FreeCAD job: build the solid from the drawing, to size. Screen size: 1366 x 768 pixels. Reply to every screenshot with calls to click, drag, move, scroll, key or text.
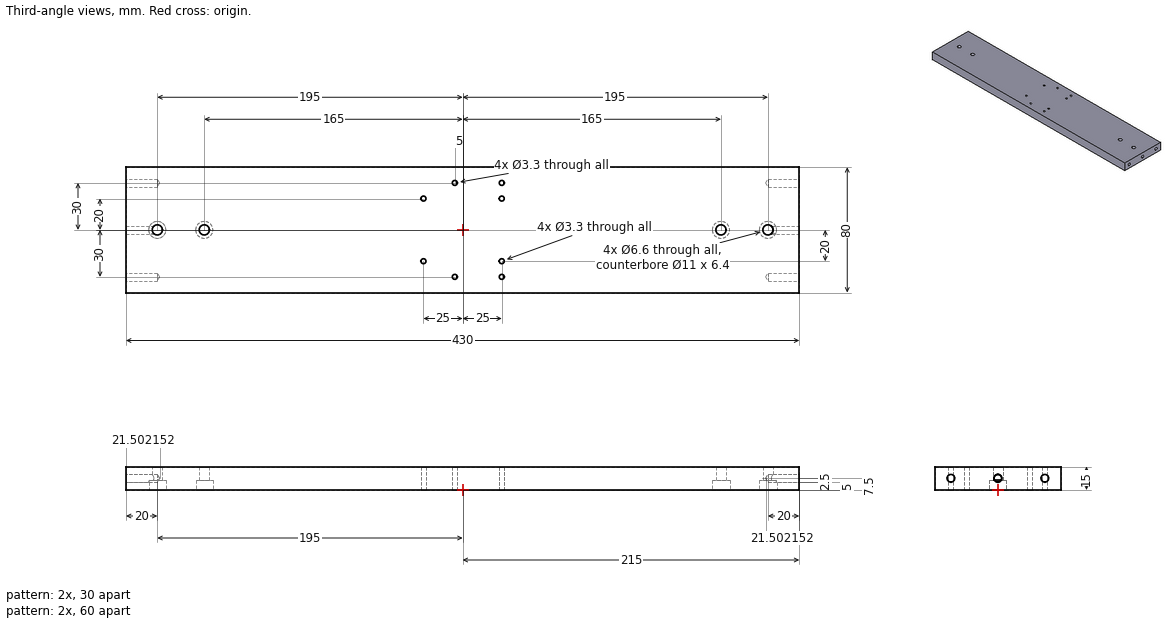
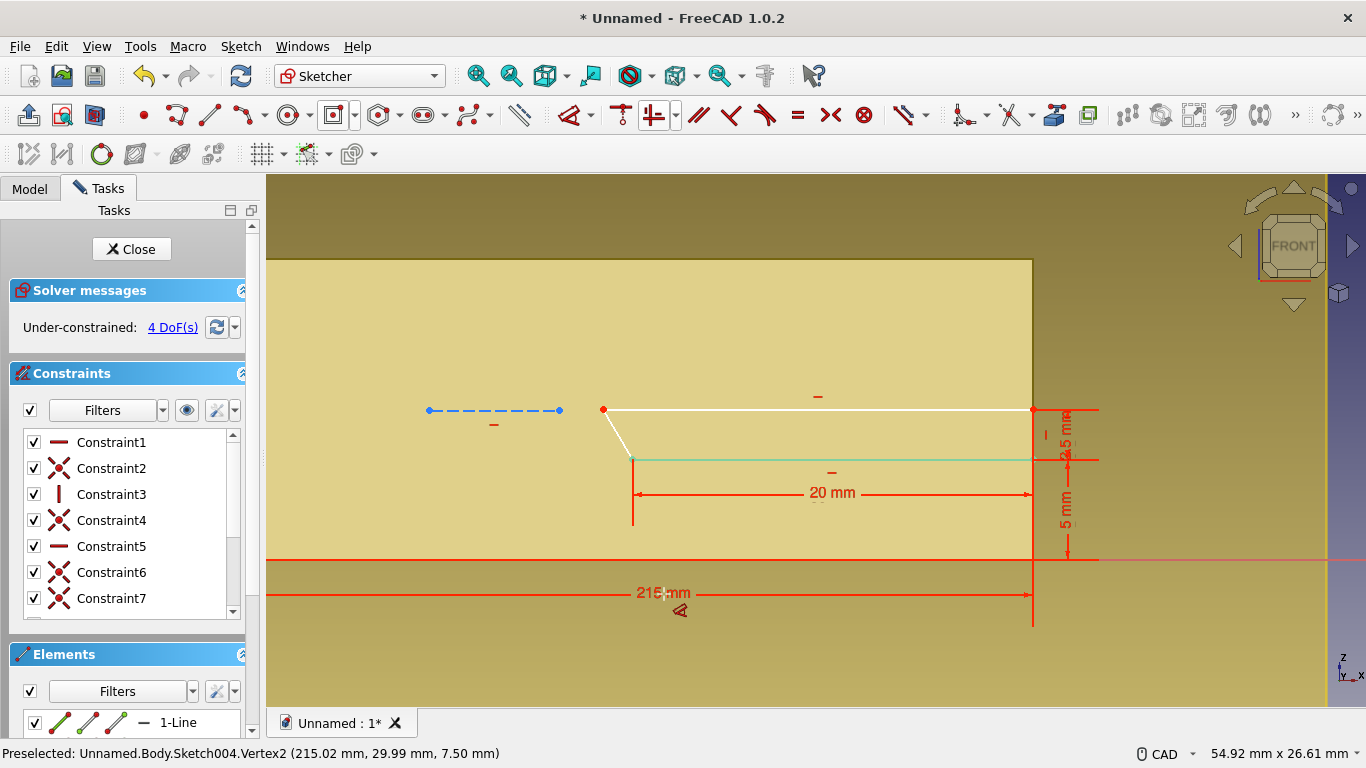
click(559, 411)
click(593, 485)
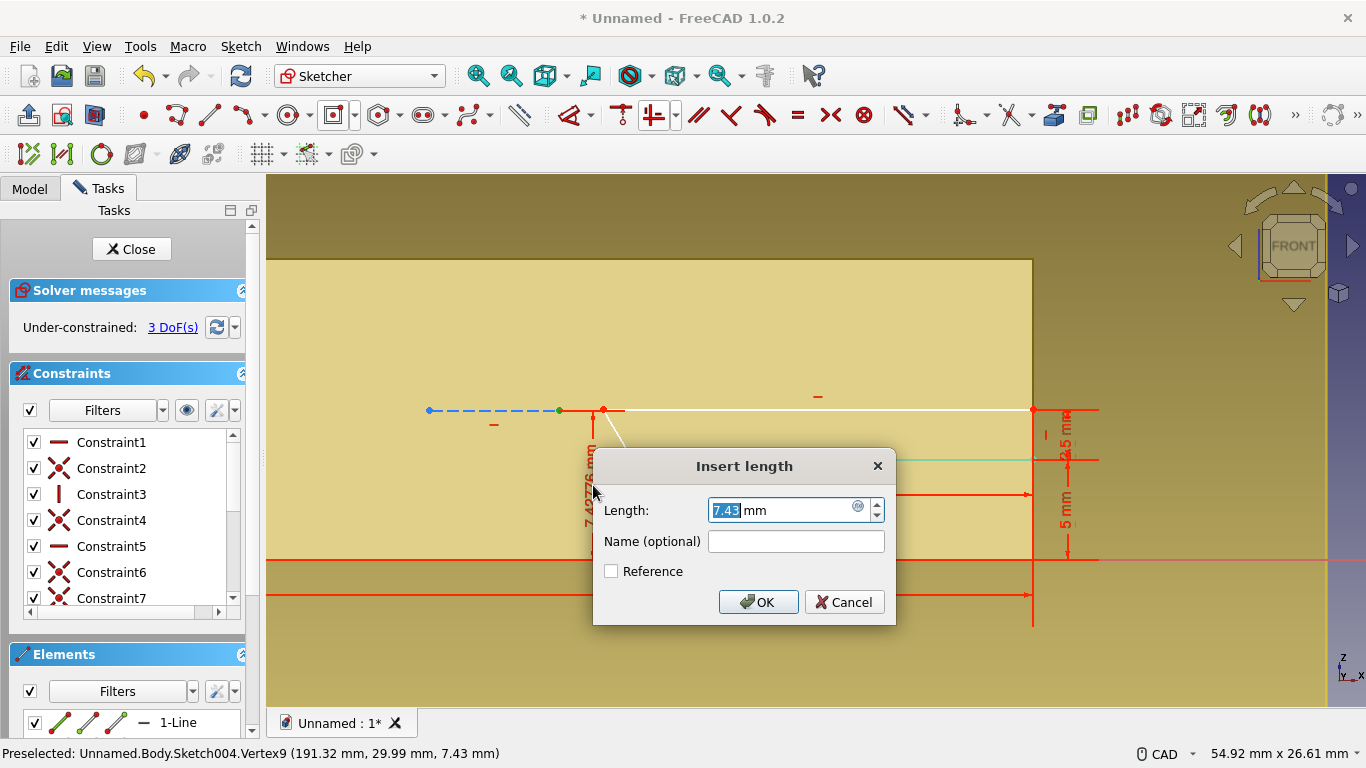
text(7.5)
key(Return)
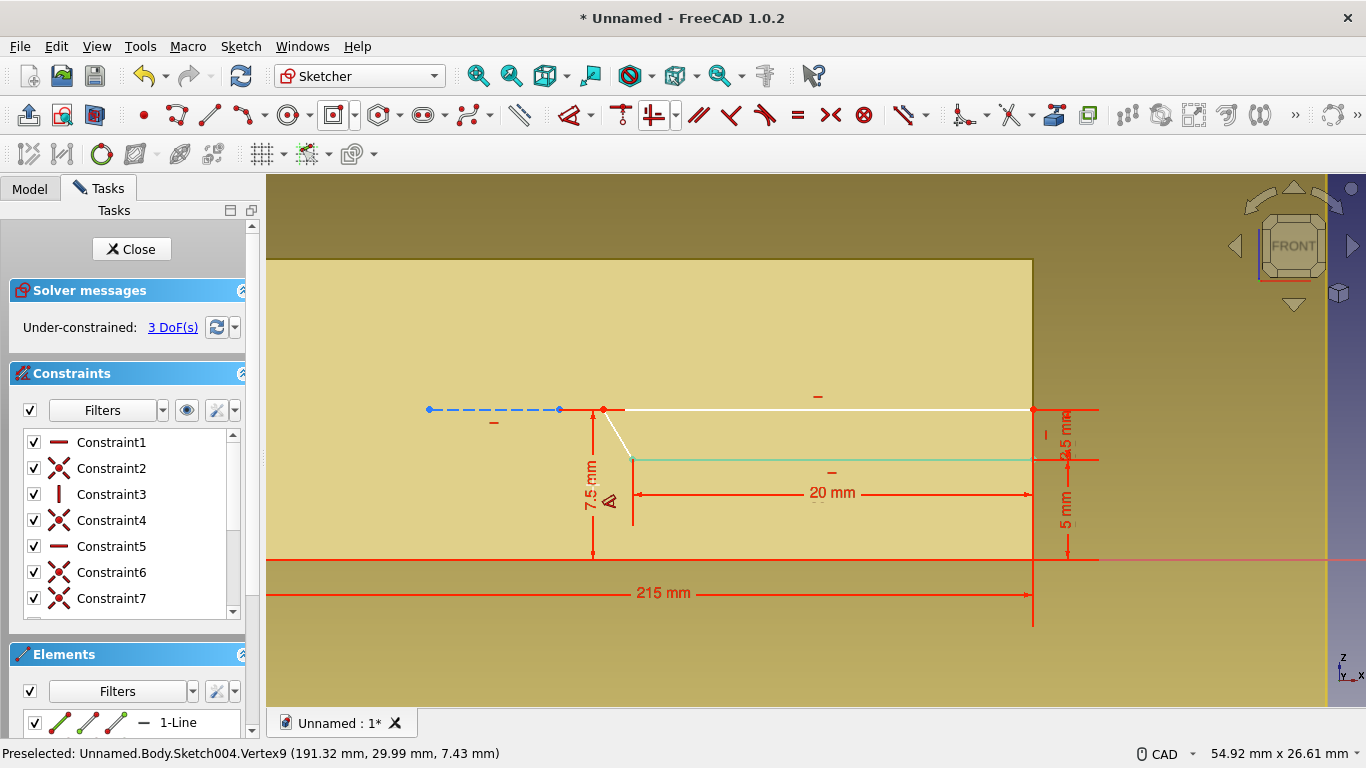
click(732, 410)
click(818, 376)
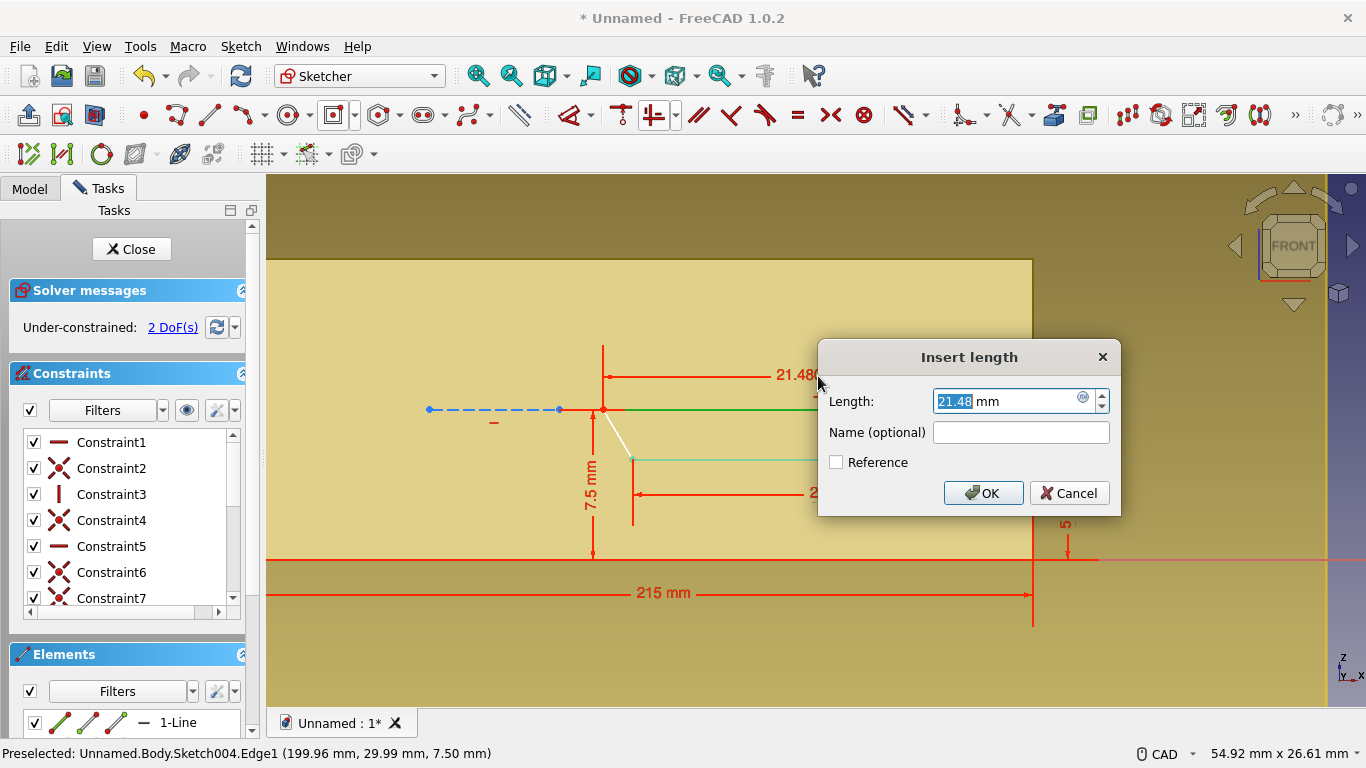
text(21.502152)
key(Return)
key(Escape)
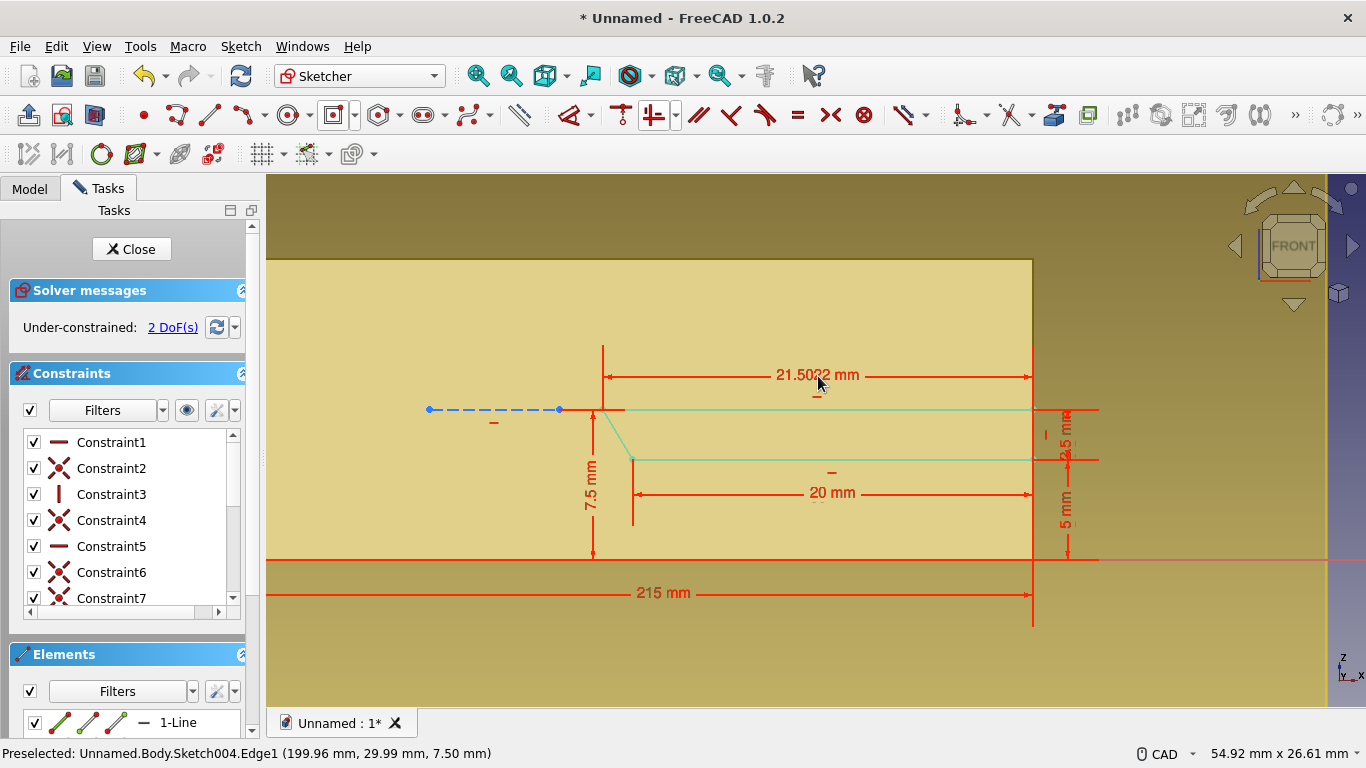
click(132, 249)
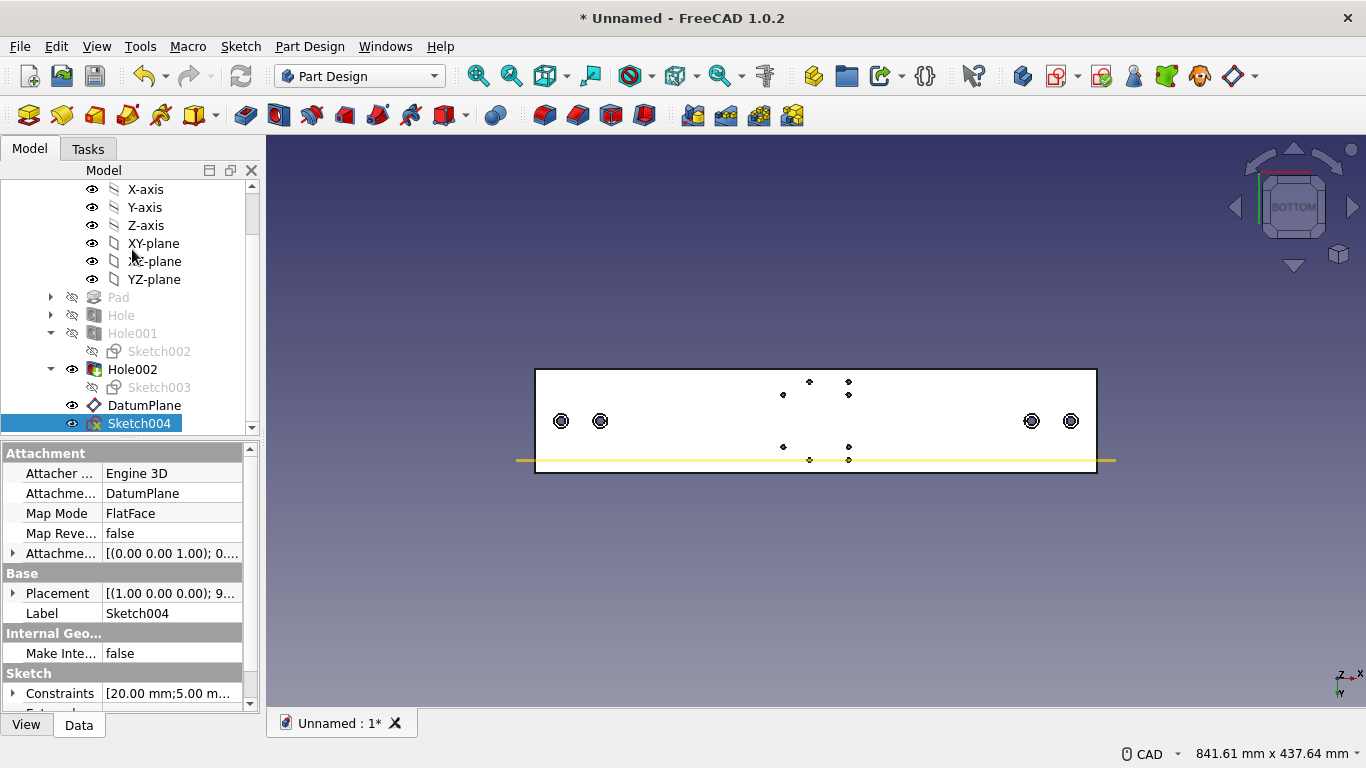
click(312, 116)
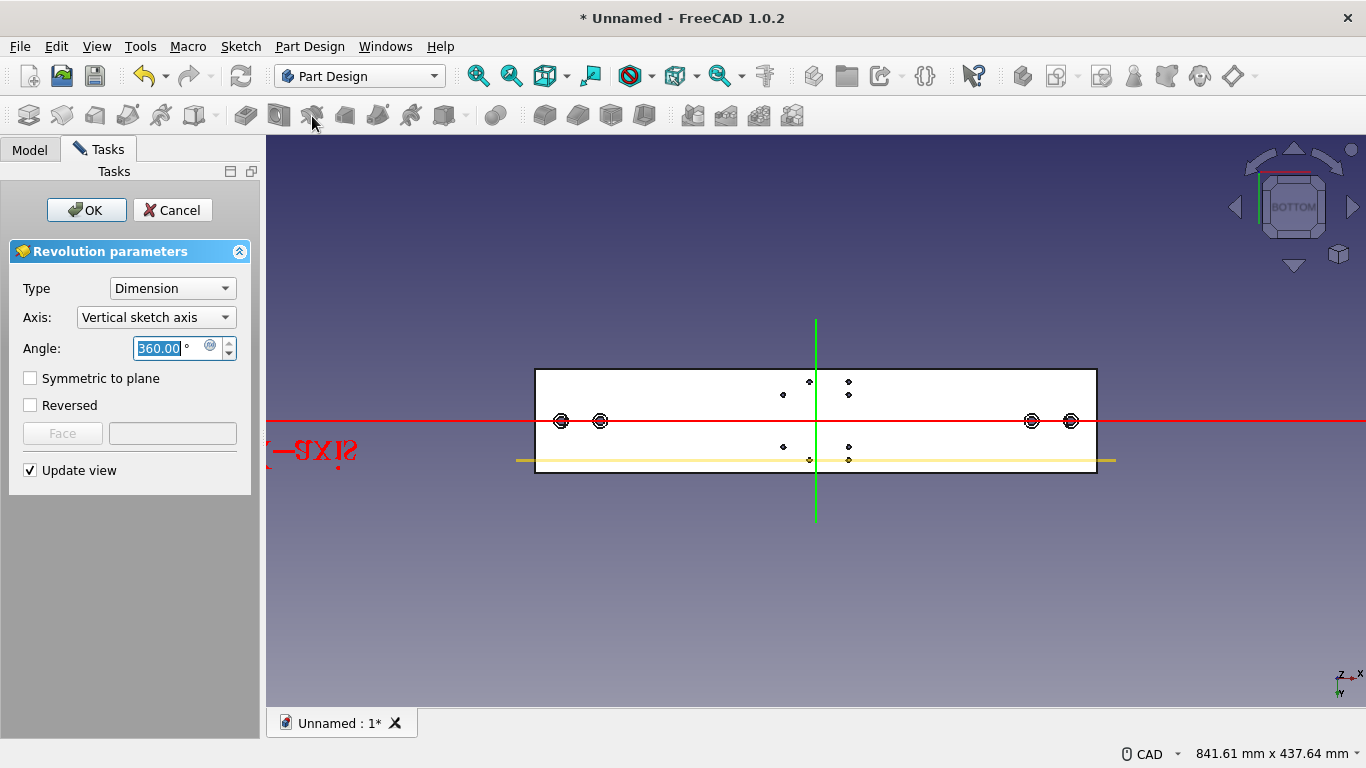
click(157, 318)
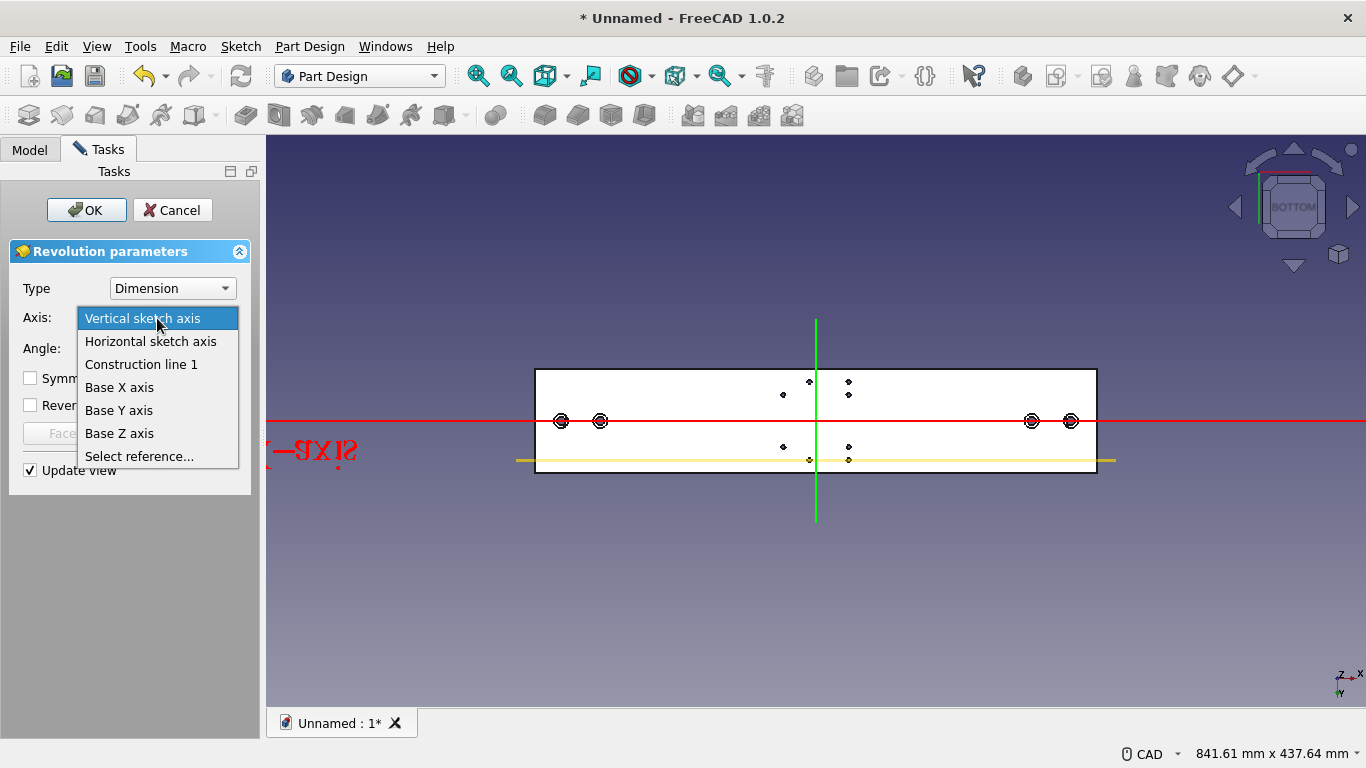
click(156, 364)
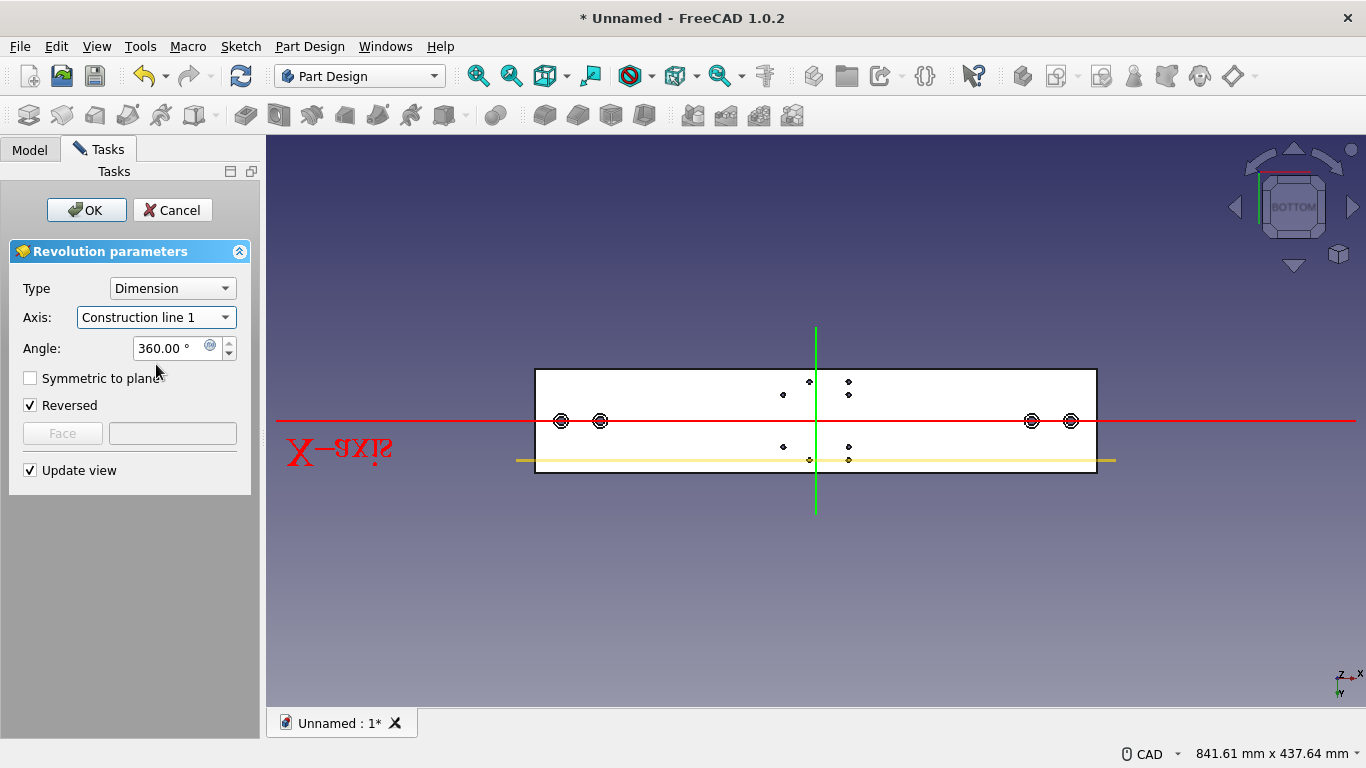
click(87, 210)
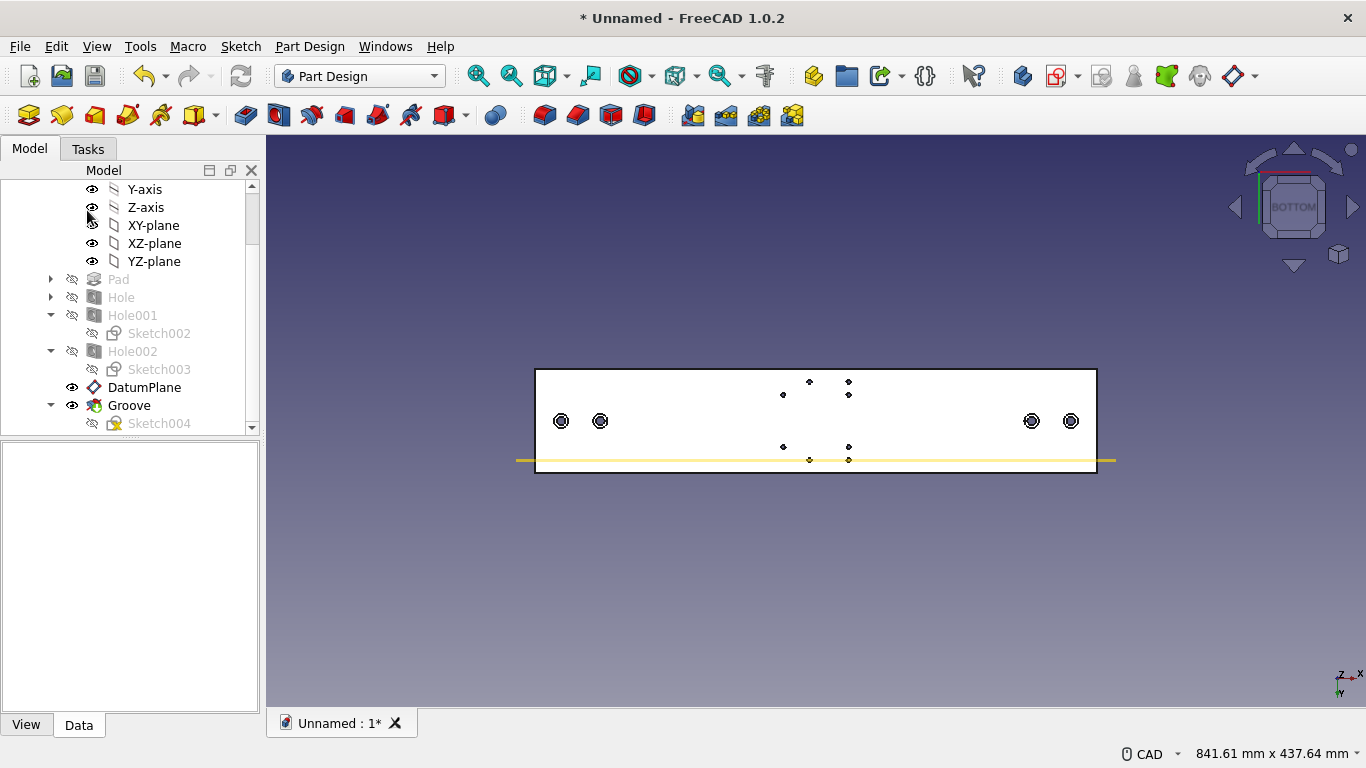
click(117, 387)
key(space)